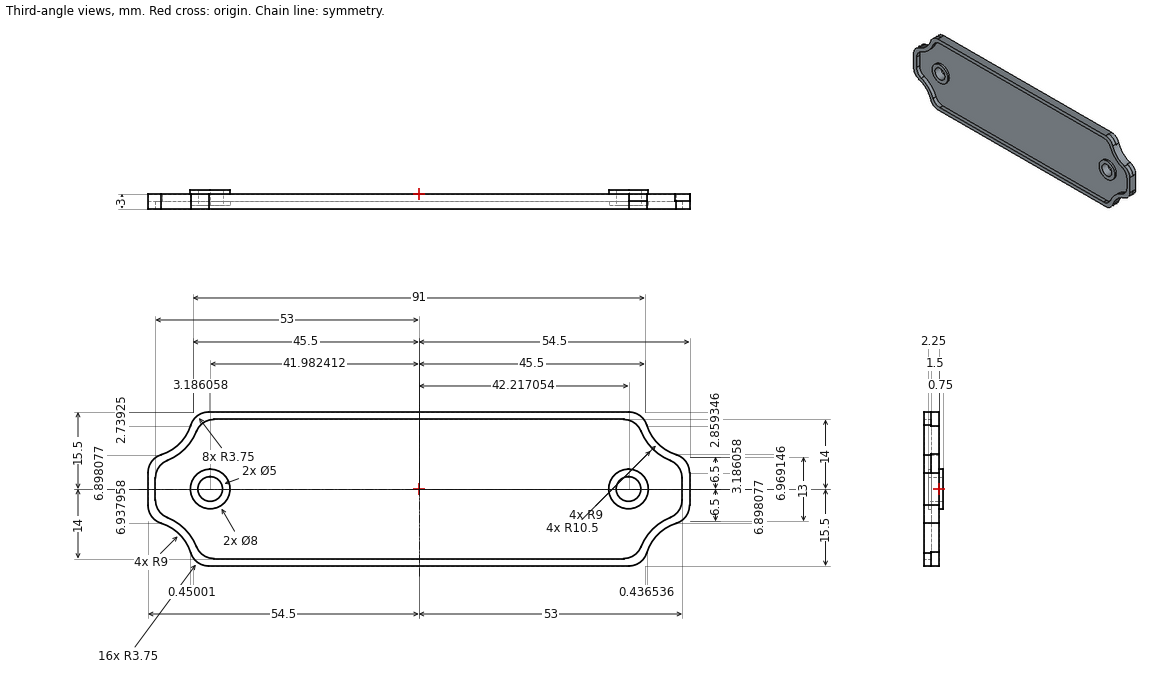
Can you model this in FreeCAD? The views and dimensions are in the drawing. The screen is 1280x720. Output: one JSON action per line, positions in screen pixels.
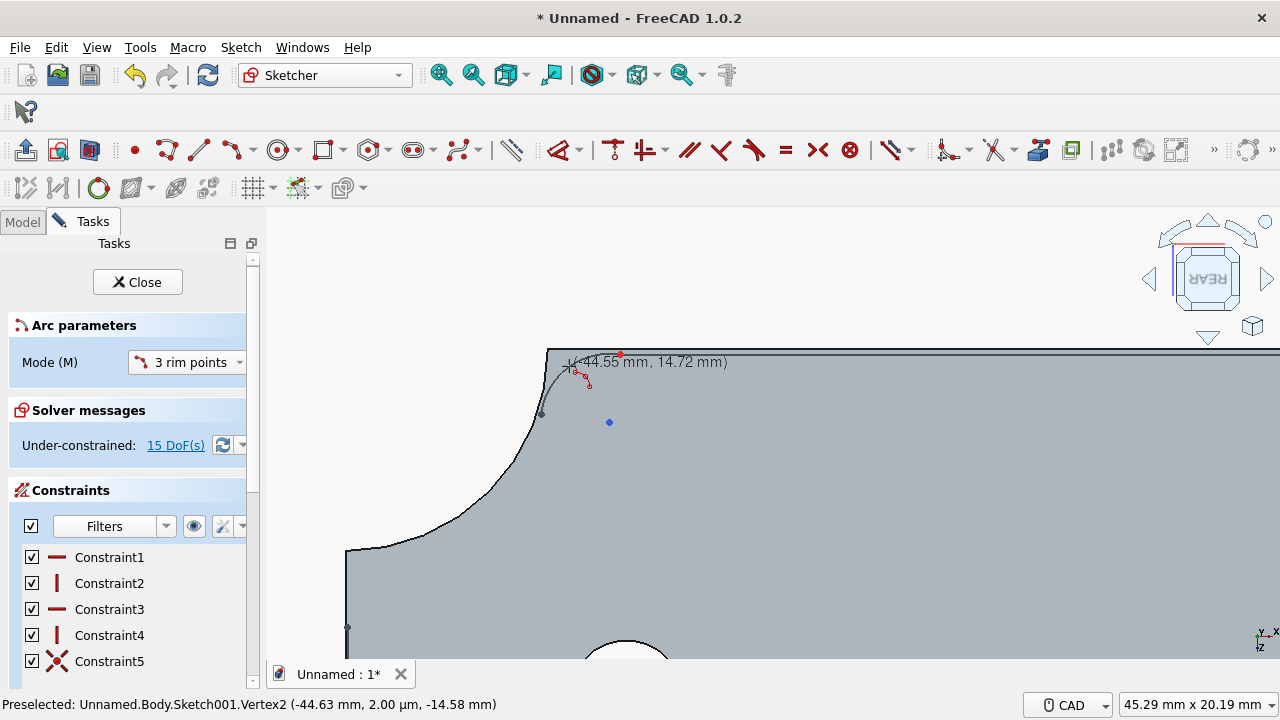
{"action": "scroll", "coordinate": [422, 347], "scroll_direction": "down", "scroll_amount": 7}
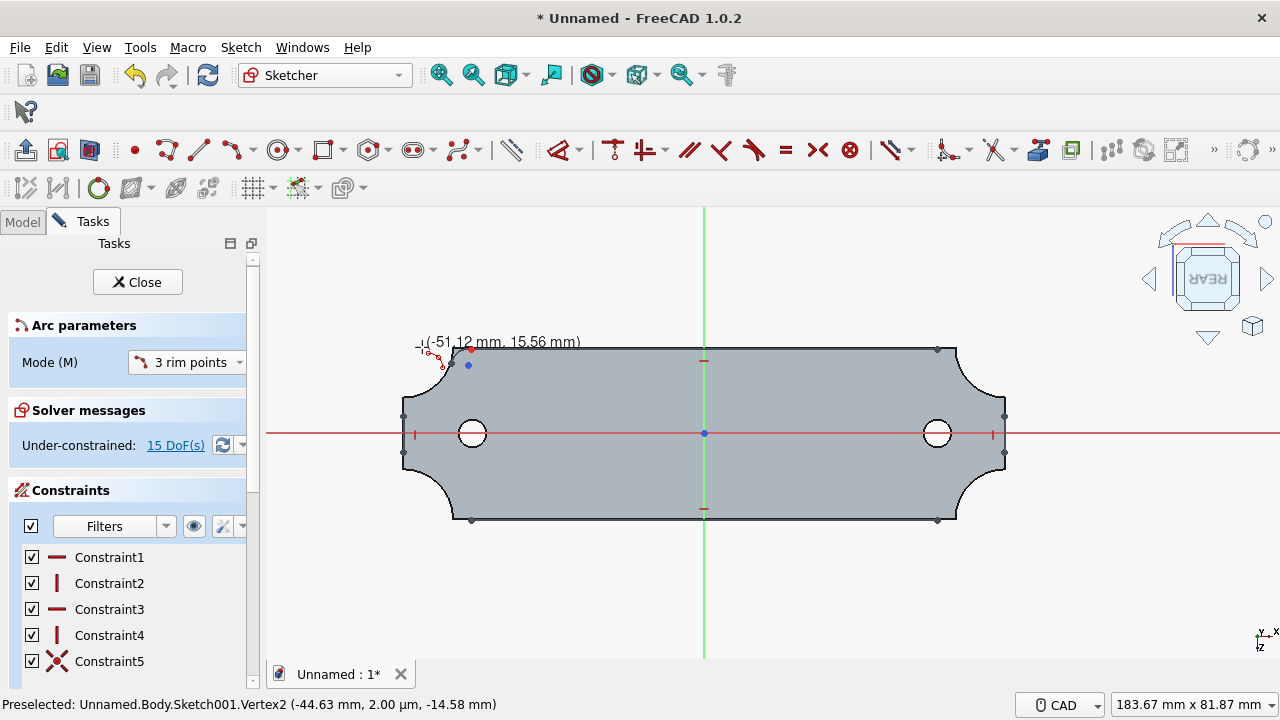
{"action": "left_click", "coordinate": [451, 364]}
{"action": "left_click", "coordinate": [418, 395]}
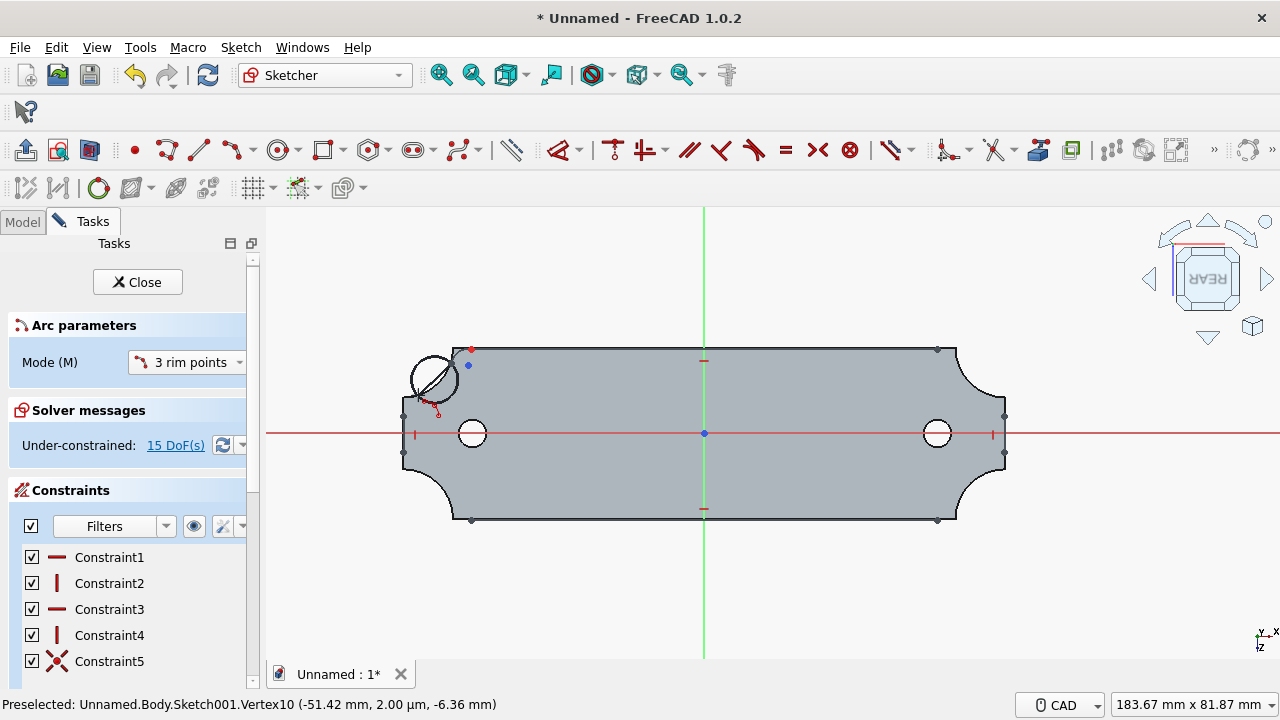
{"action": "scroll", "coordinate": [439, 383], "scroll_direction": "up", "scroll_amount": 6}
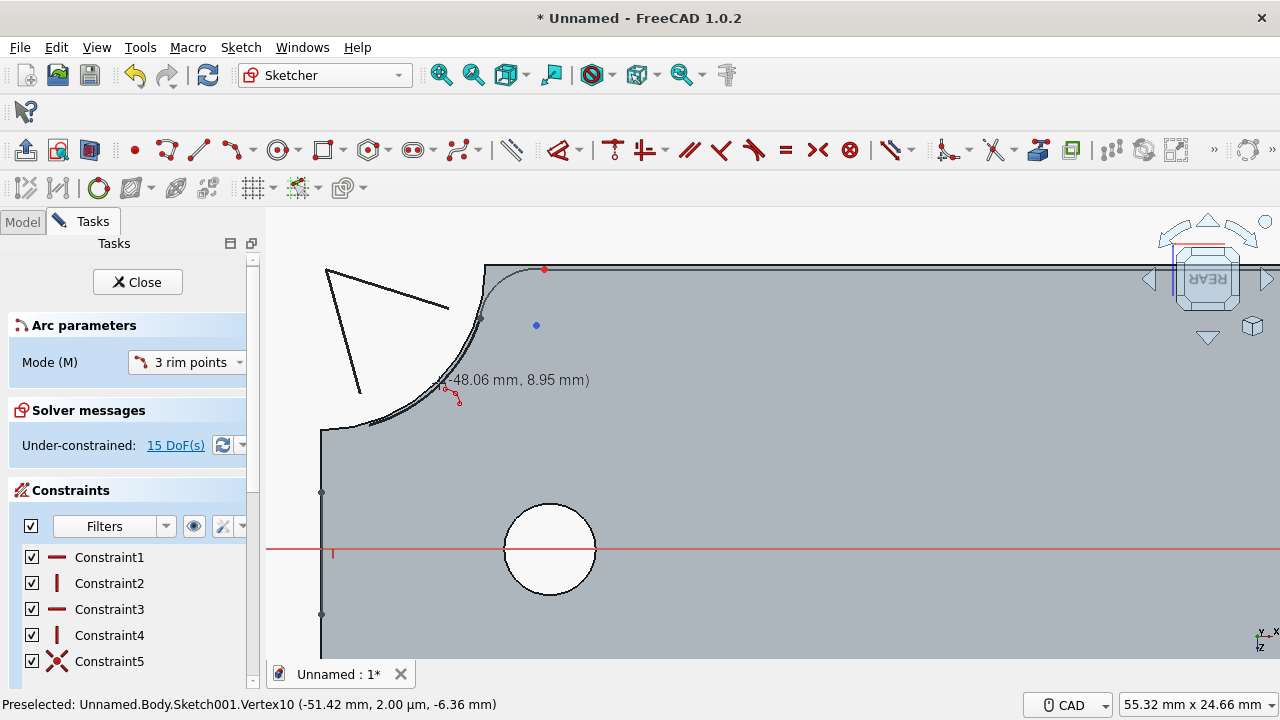
{"action": "left_click", "coordinate": [437, 382]}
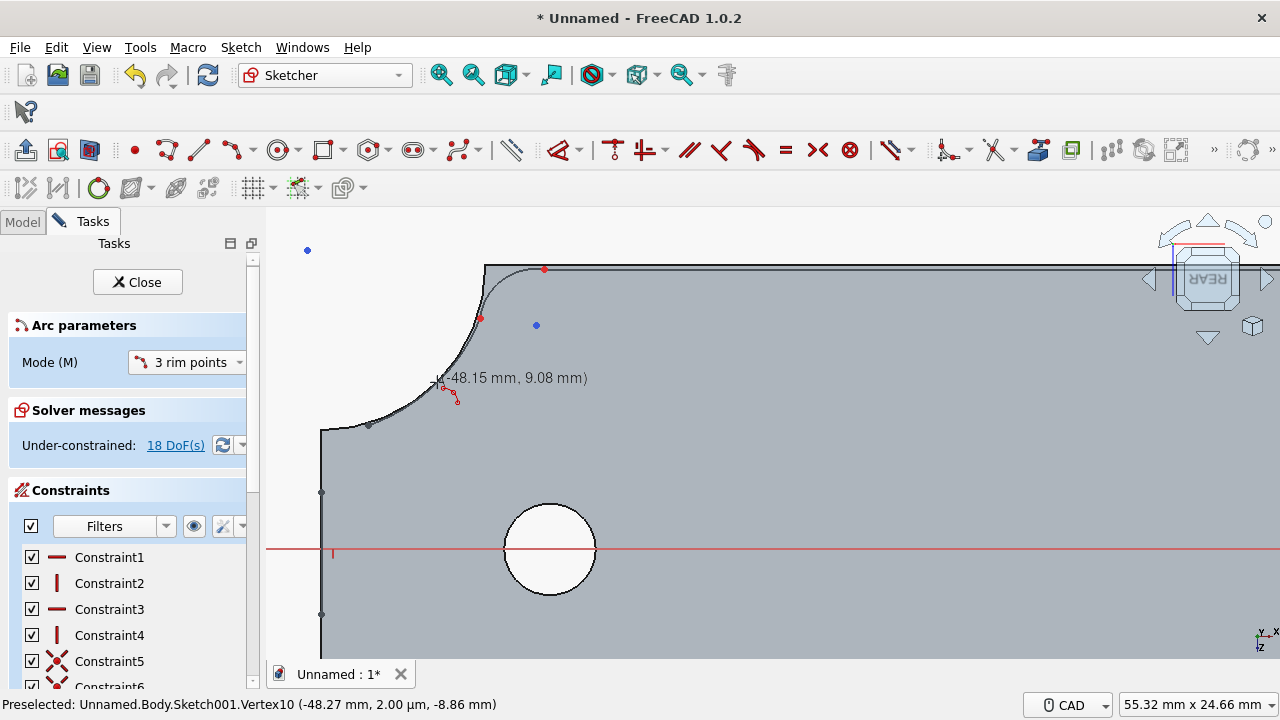
{"action": "scroll", "coordinate": [439, 383], "scroll_direction": "down", "scroll_amount": 6}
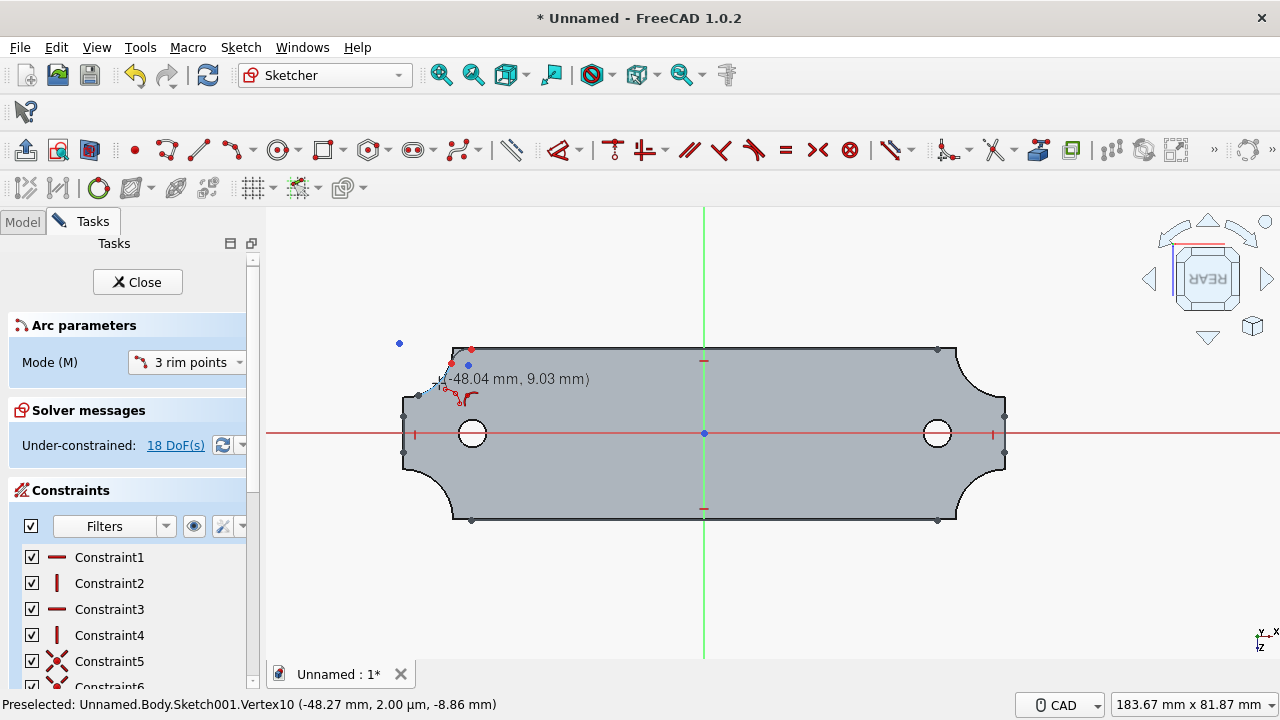
{"action": "left_click", "coordinate": [418, 396]}
{"action": "left_click", "coordinate": [404, 416]}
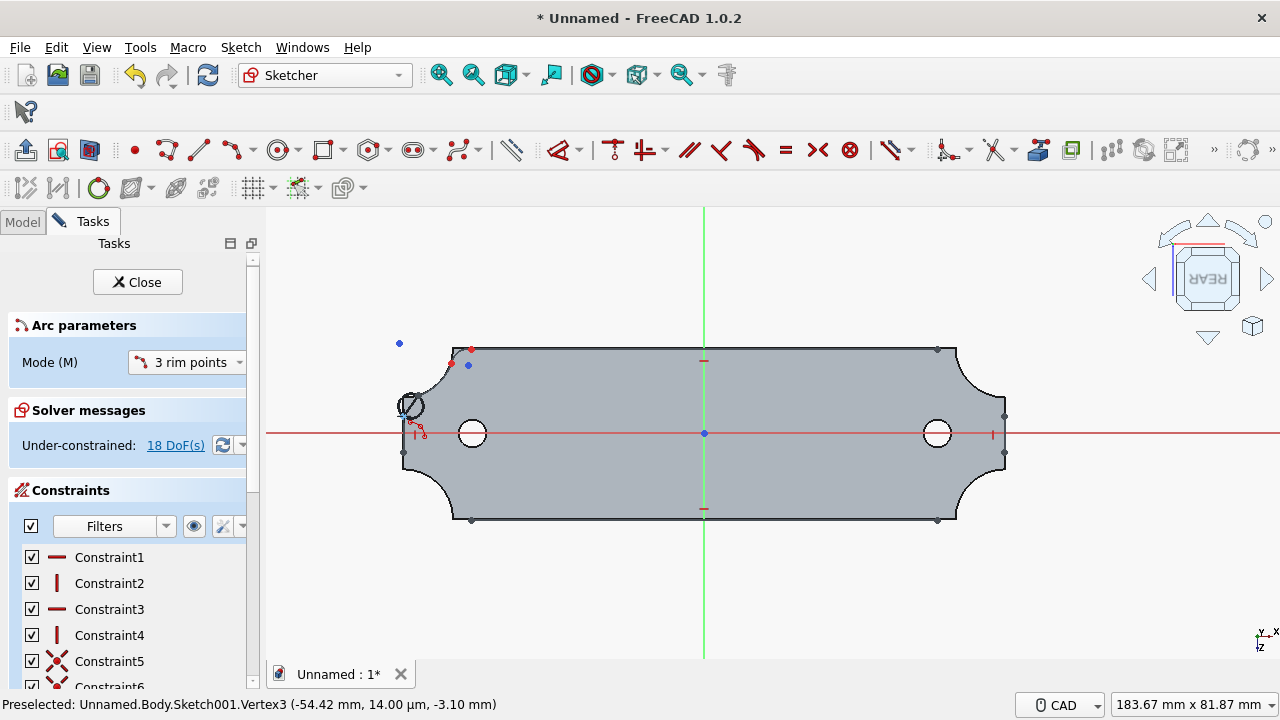
{"action": "scroll", "coordinate": [407, 403], "scroll_direction": "up", "scroll_amount": 7}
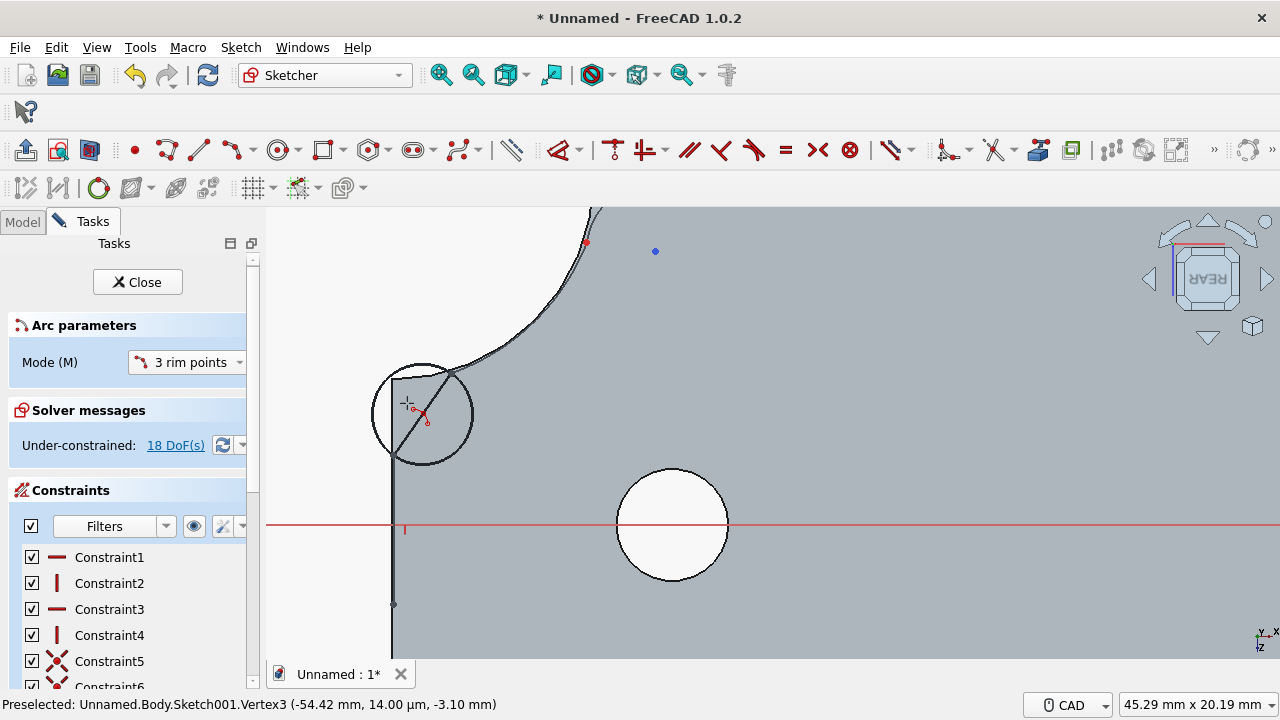
{"action": "left_click", "coordinate": [409, 401]}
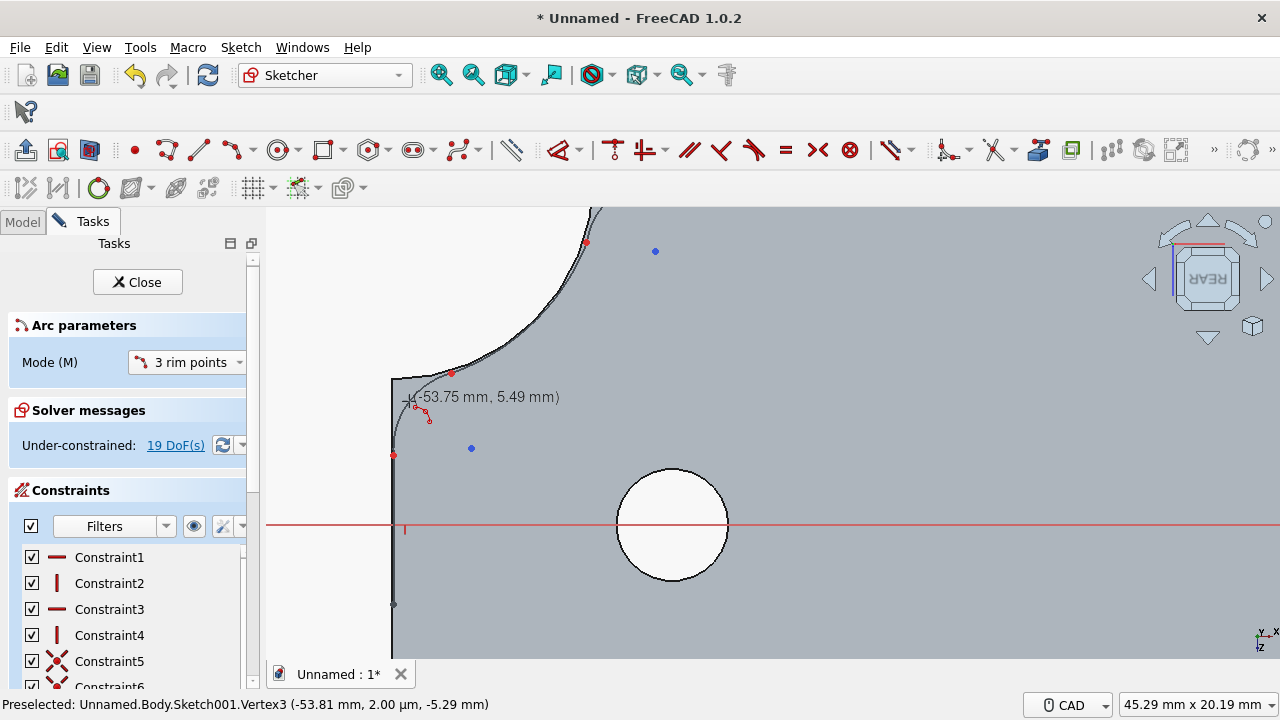
{"action": "scroll", "coordinate": [407, 403], "scroll_direction": "down", "scroll_amount": 7}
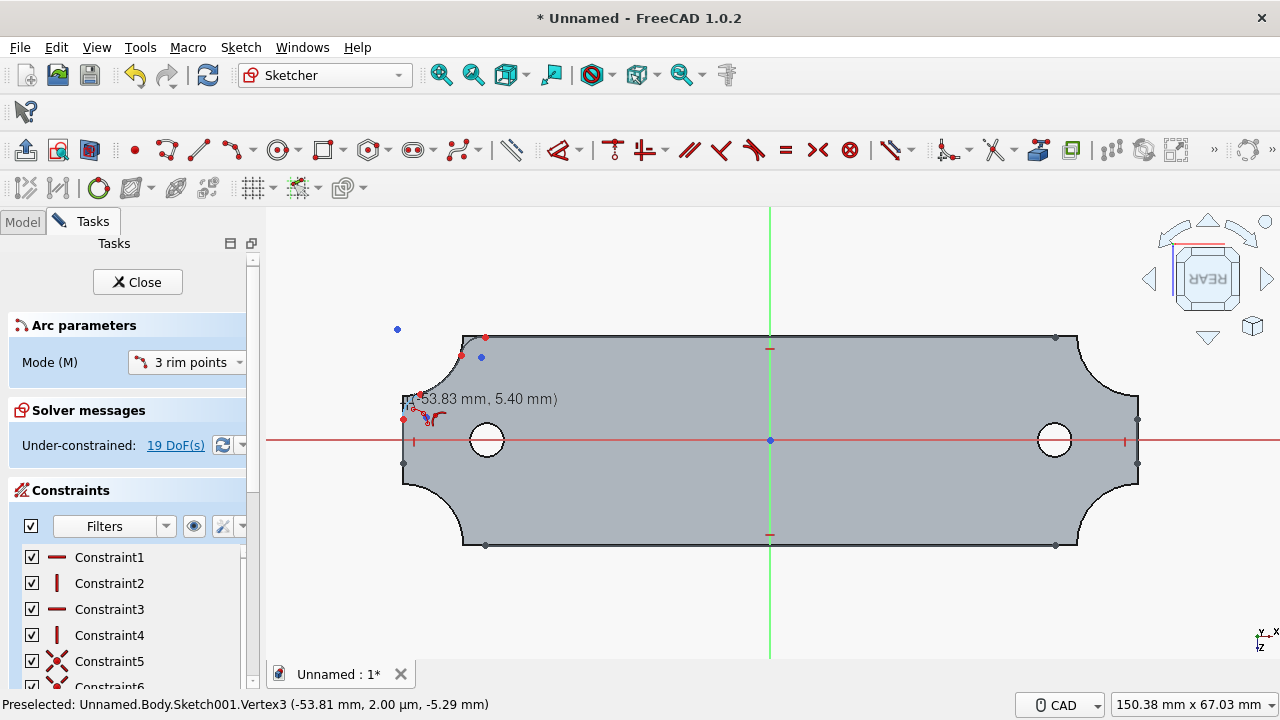
{"action": "left_click", "coordinate": [404, 453]}
{"action": "left_click", "coordinate": [418, 471]}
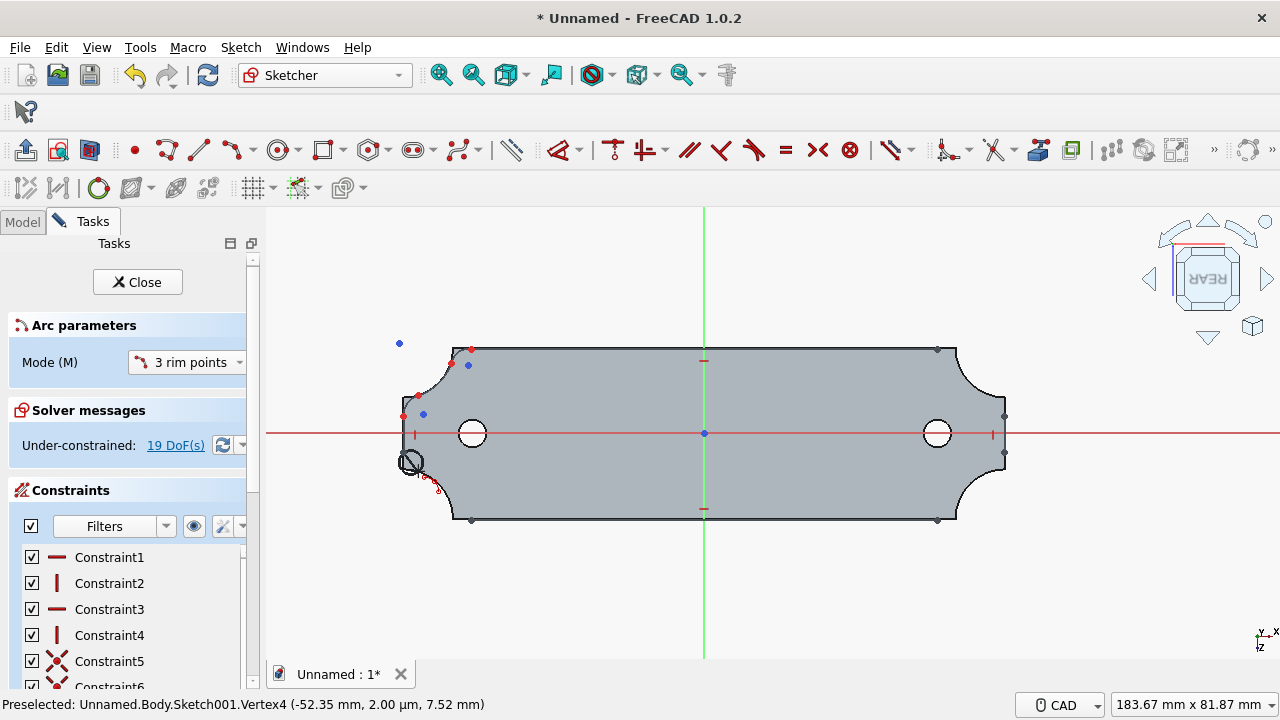
{"action": "scroll", "coordinate": [407, 464], "scroll_direction": "up", "scroll_amount": 7}